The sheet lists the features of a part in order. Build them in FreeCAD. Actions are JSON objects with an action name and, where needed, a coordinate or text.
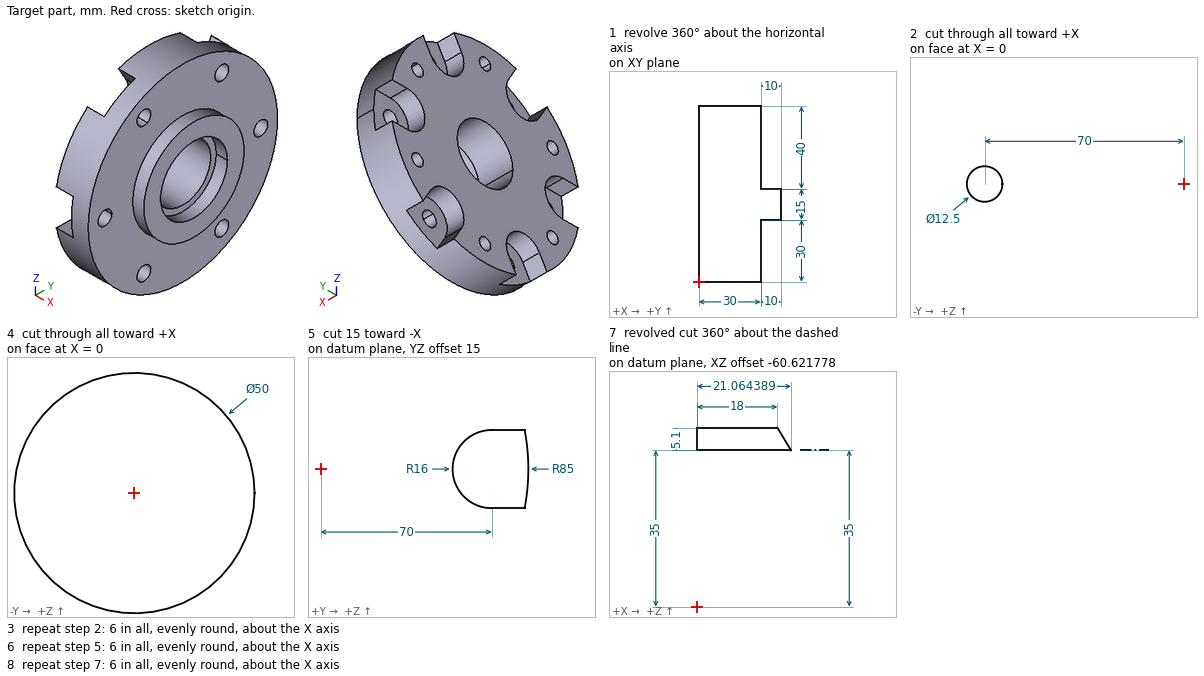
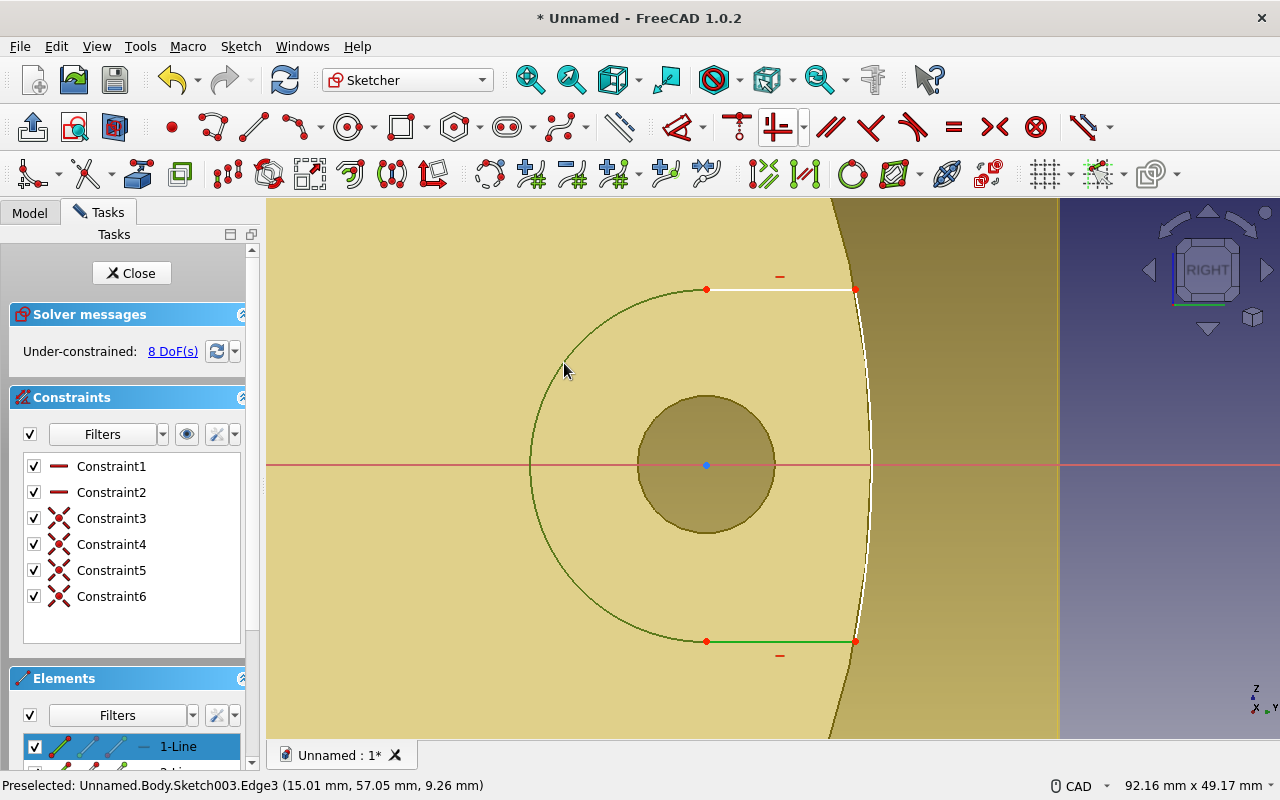
{"action": "left_click", "coordinate": [913, 128]}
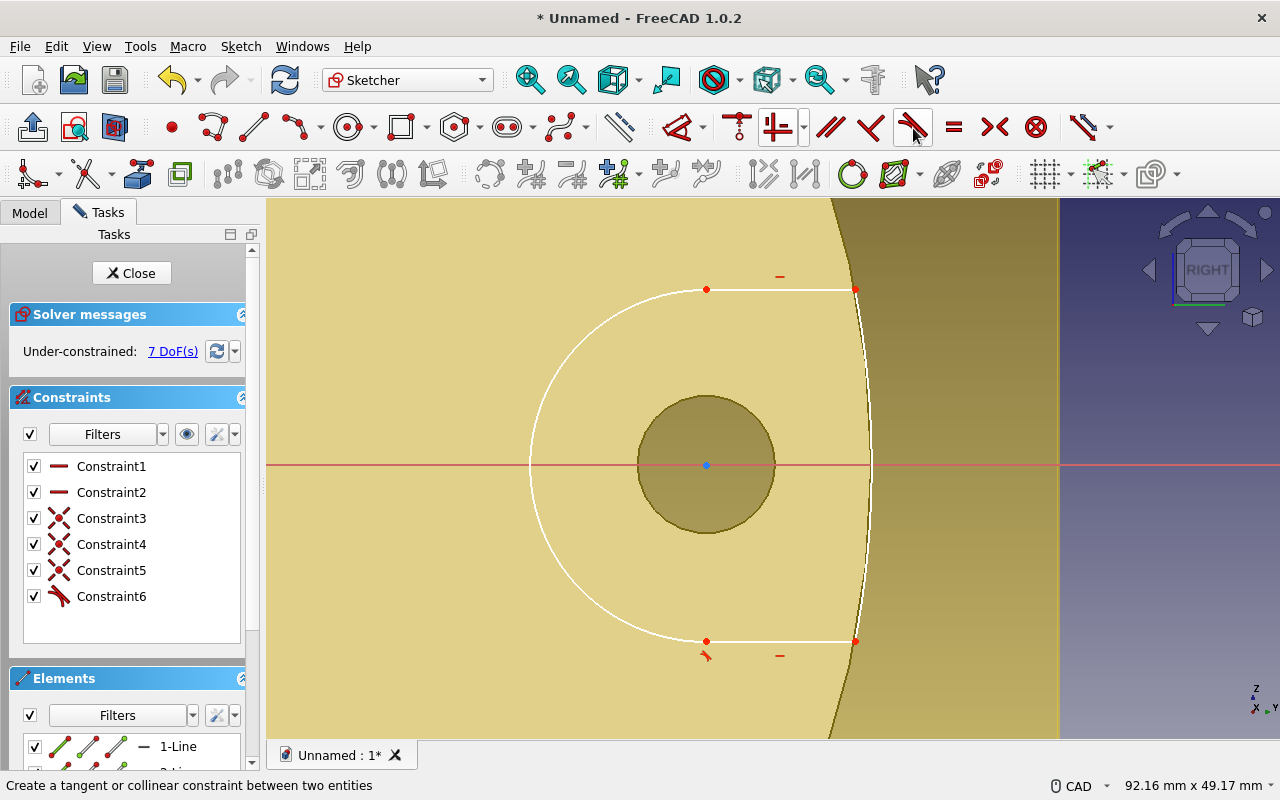
{"action": "left_click", "coordinate": [751, 290]}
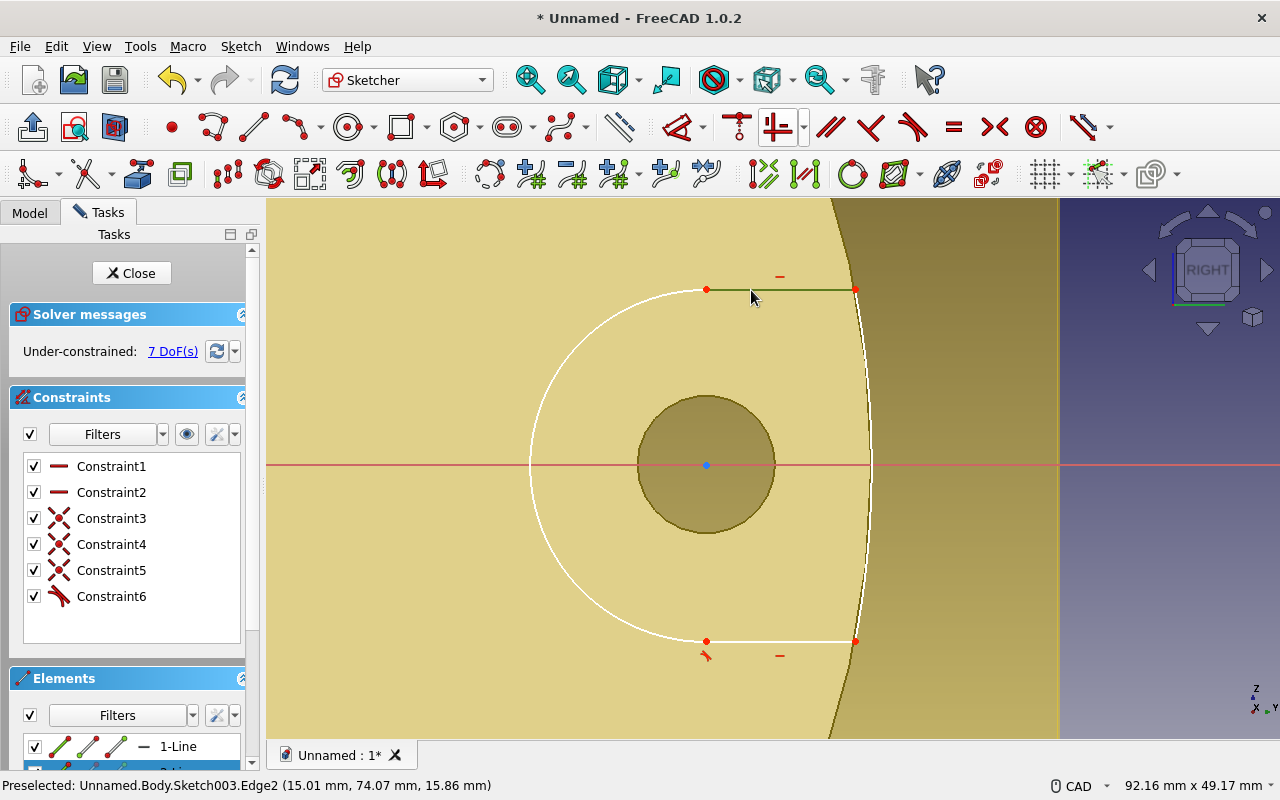
{"action": "left_click", "coordinate": [564, 363]}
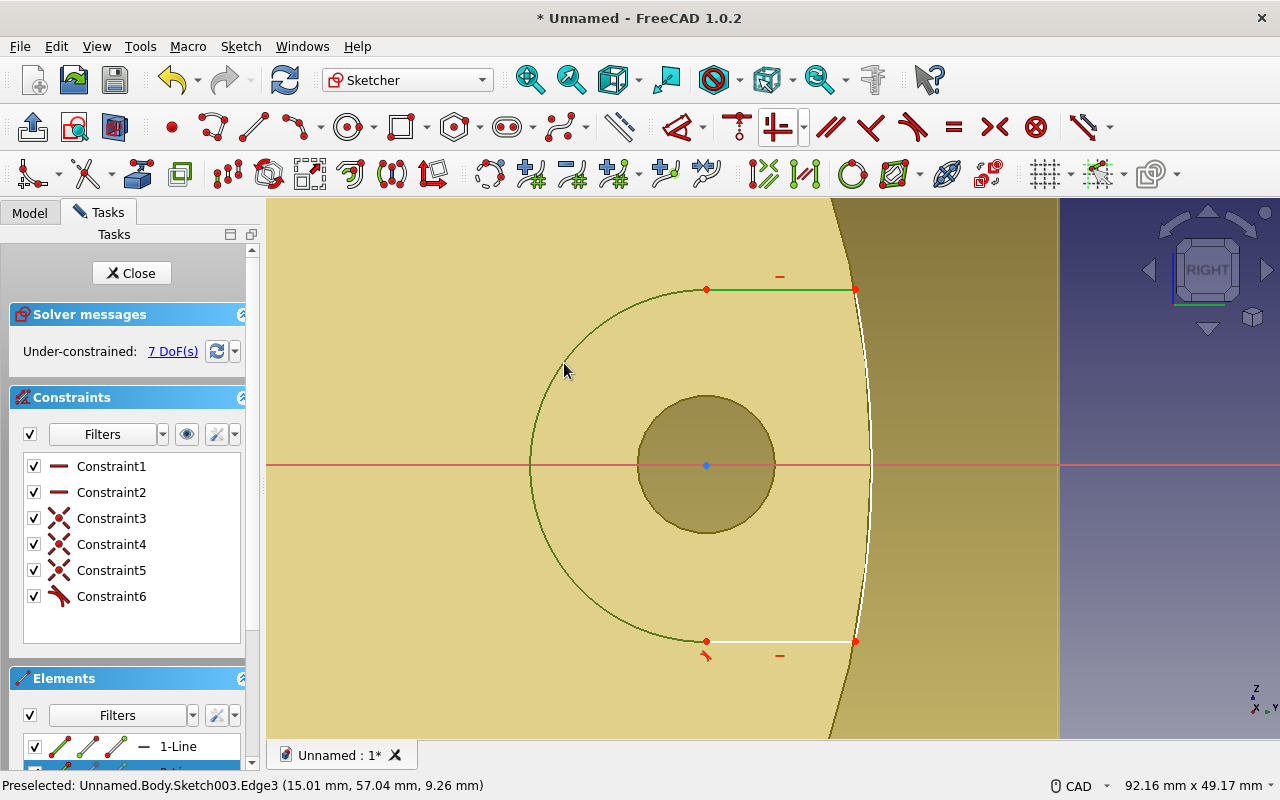
{"action": "left_click", "coordinate": [913, 128]}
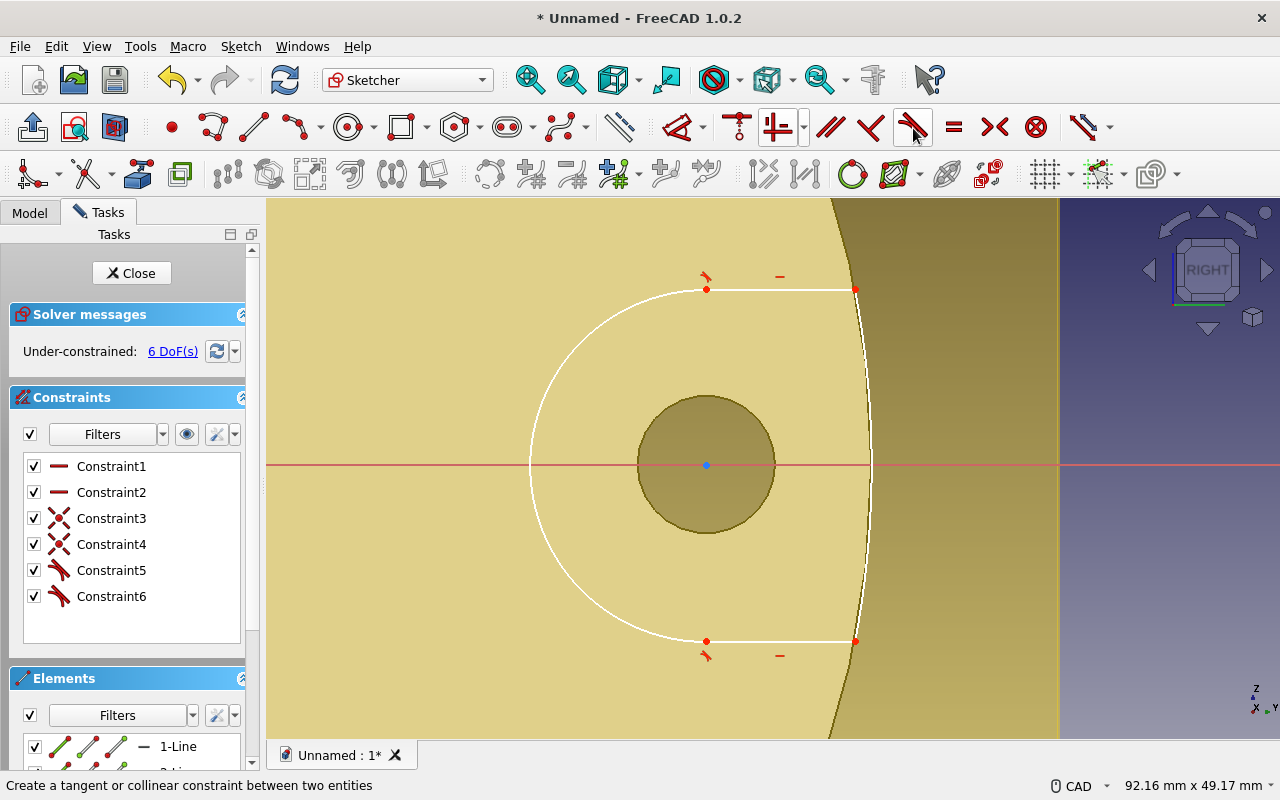
{"action": "scroll", "coordinate": [1115, 477], "scroll_direction": "down", "scroll_amount": 2}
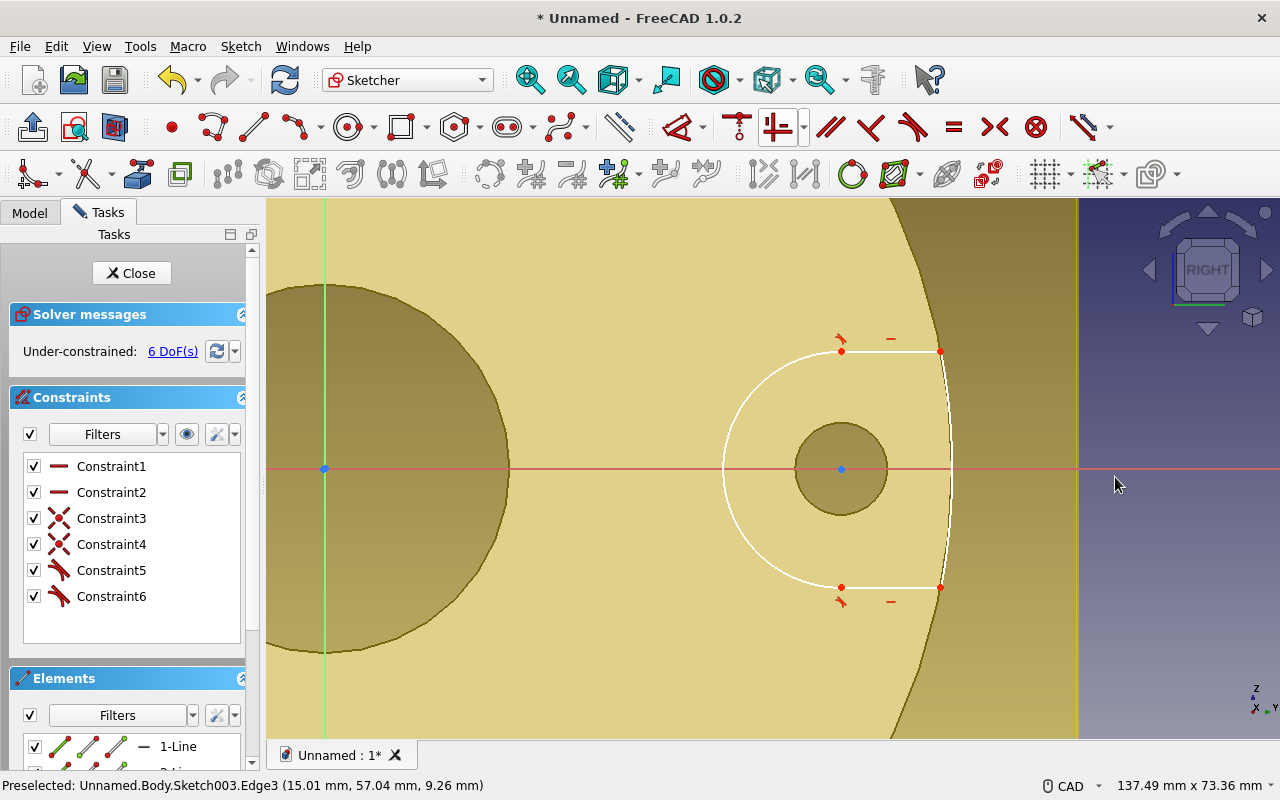
{"action": "left_click_drag", "start_coordinate": [313, 459], "coordinate": [335, 480]}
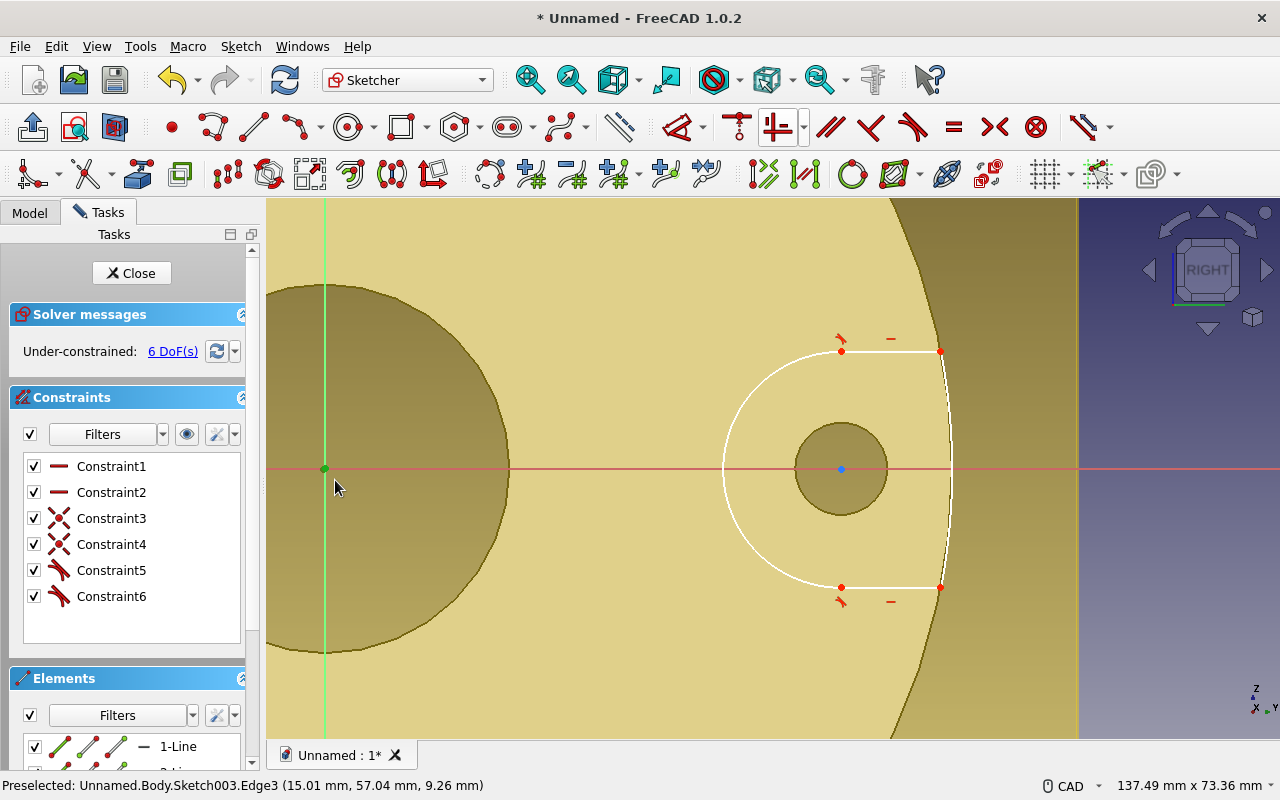
{"action": "left_click", "coordinate": [737, 128]}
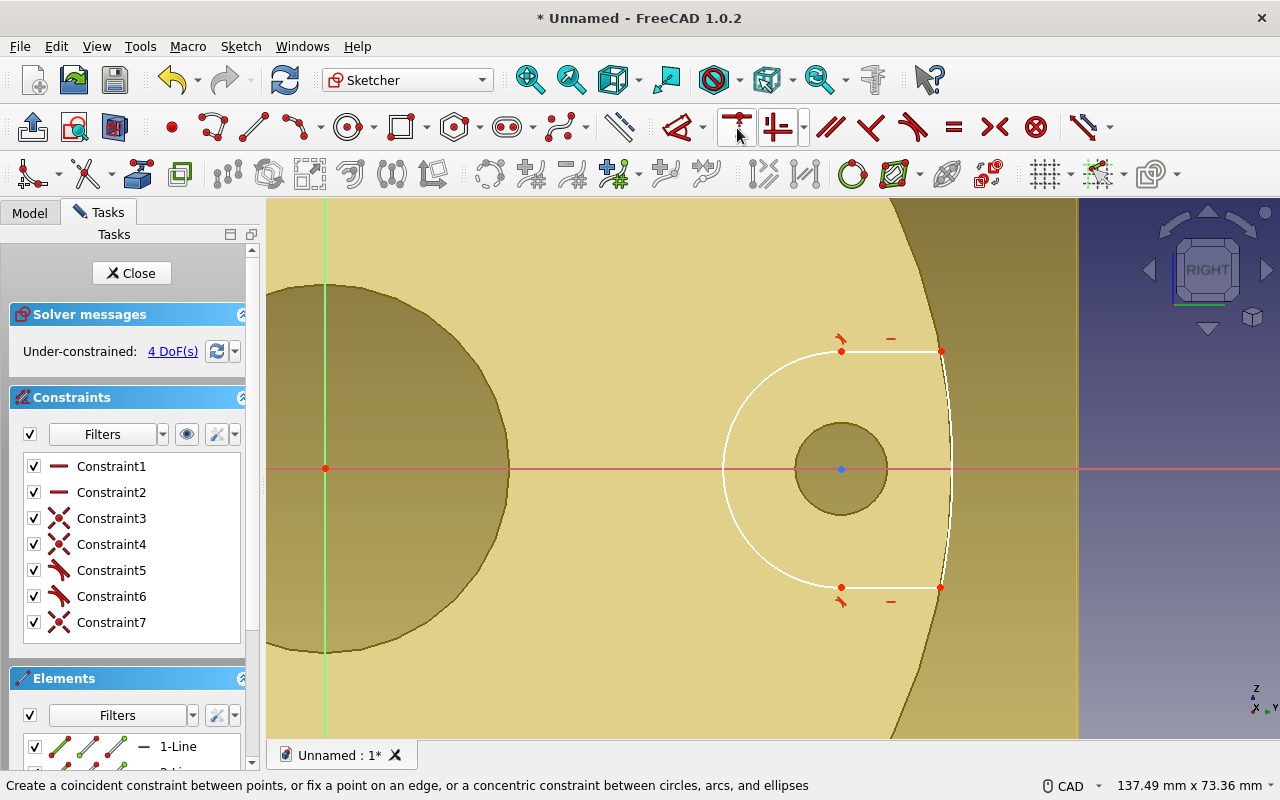
{"action": "left_click", "coordinate": [841, 470]}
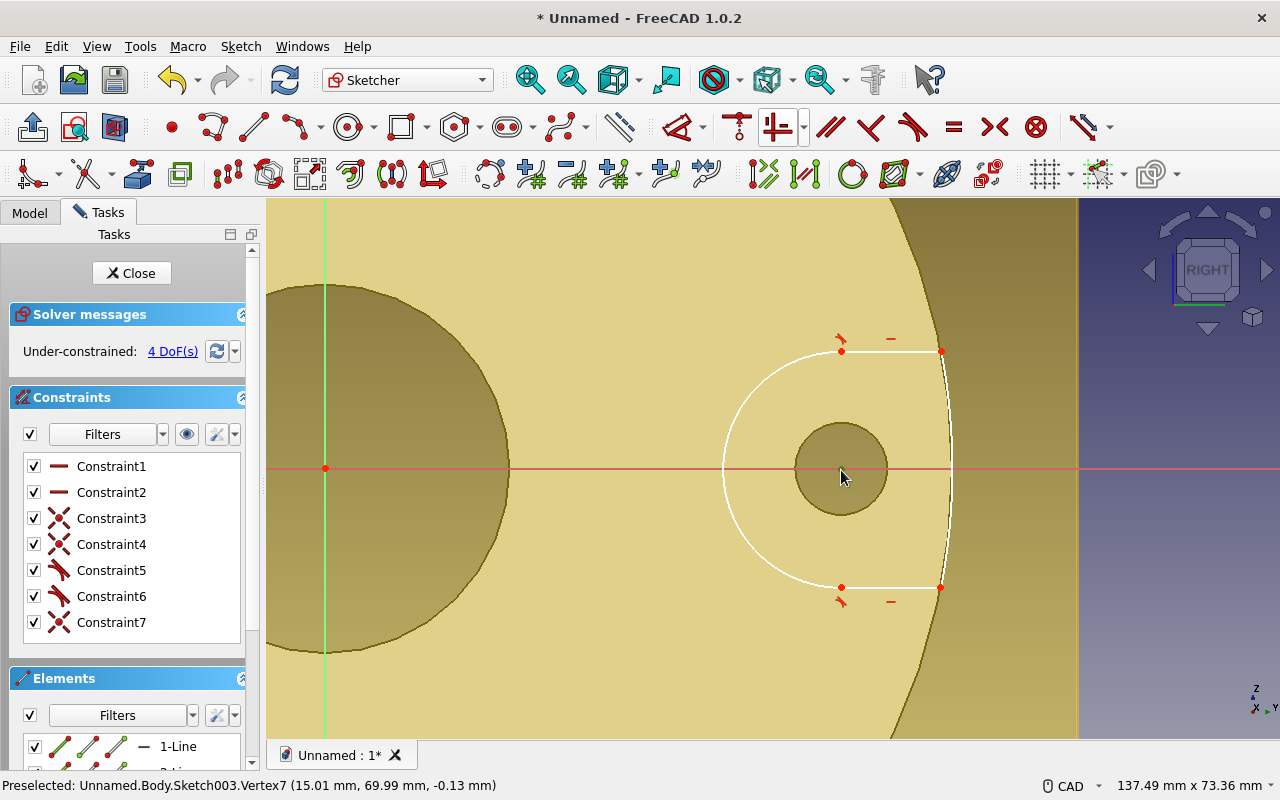
{"action": "left_click", "coordinate": [411, 469]}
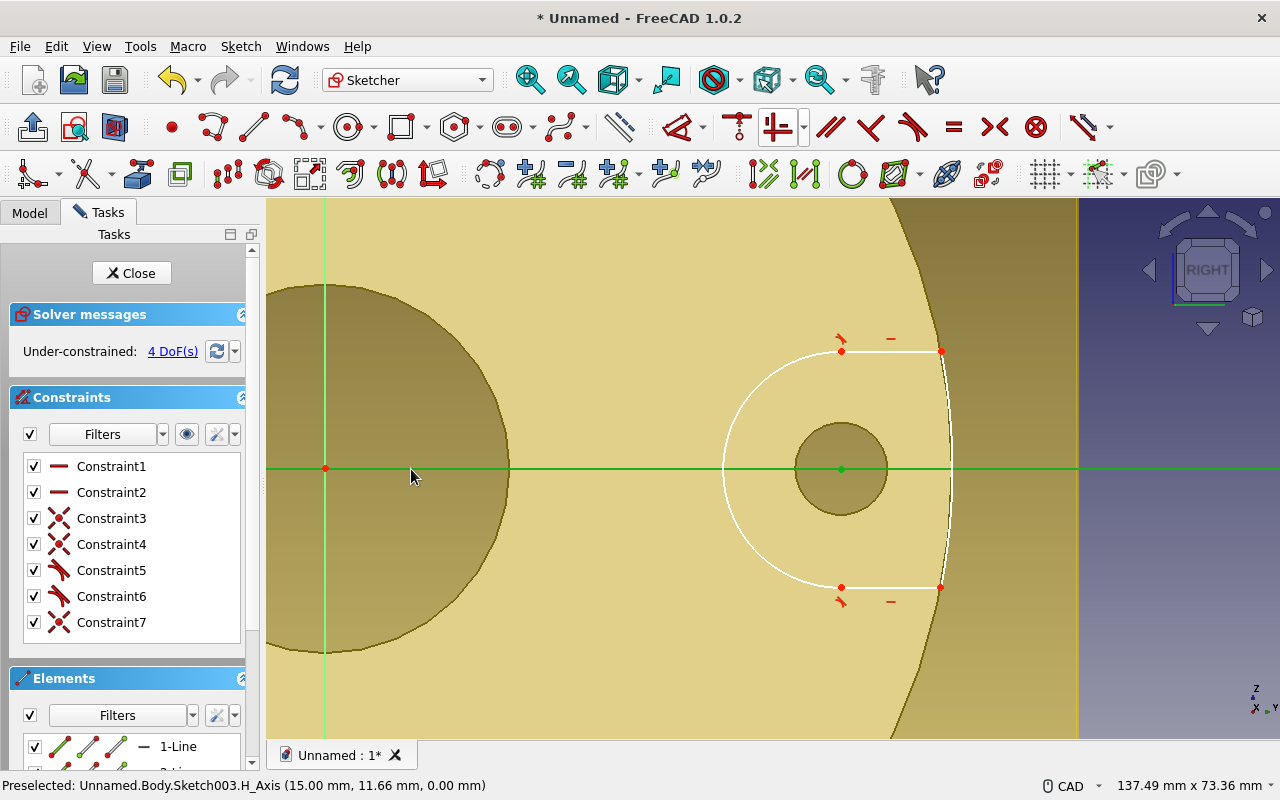
{"action": "left_click", "coordinate": [737, 128]}